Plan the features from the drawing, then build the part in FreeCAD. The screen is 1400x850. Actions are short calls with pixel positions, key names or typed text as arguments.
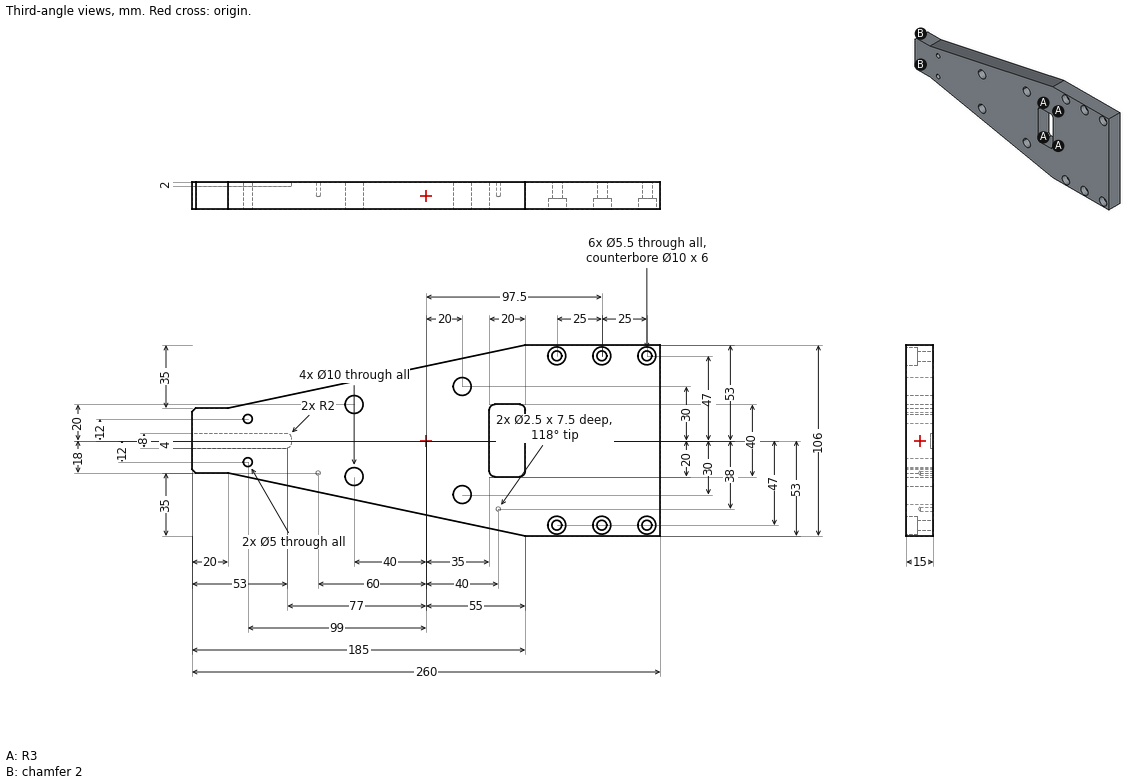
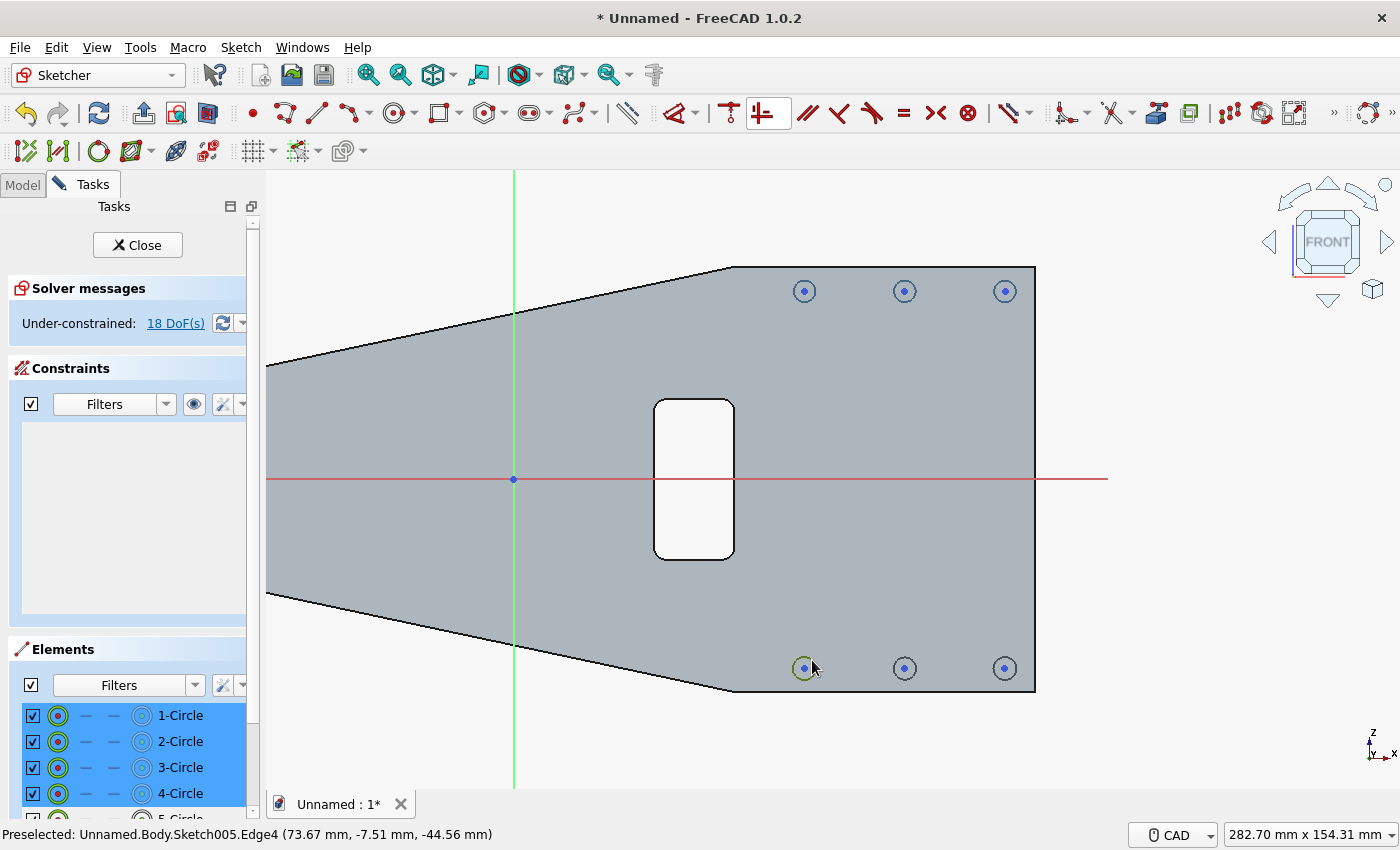
scroll(913, 661, up, 2)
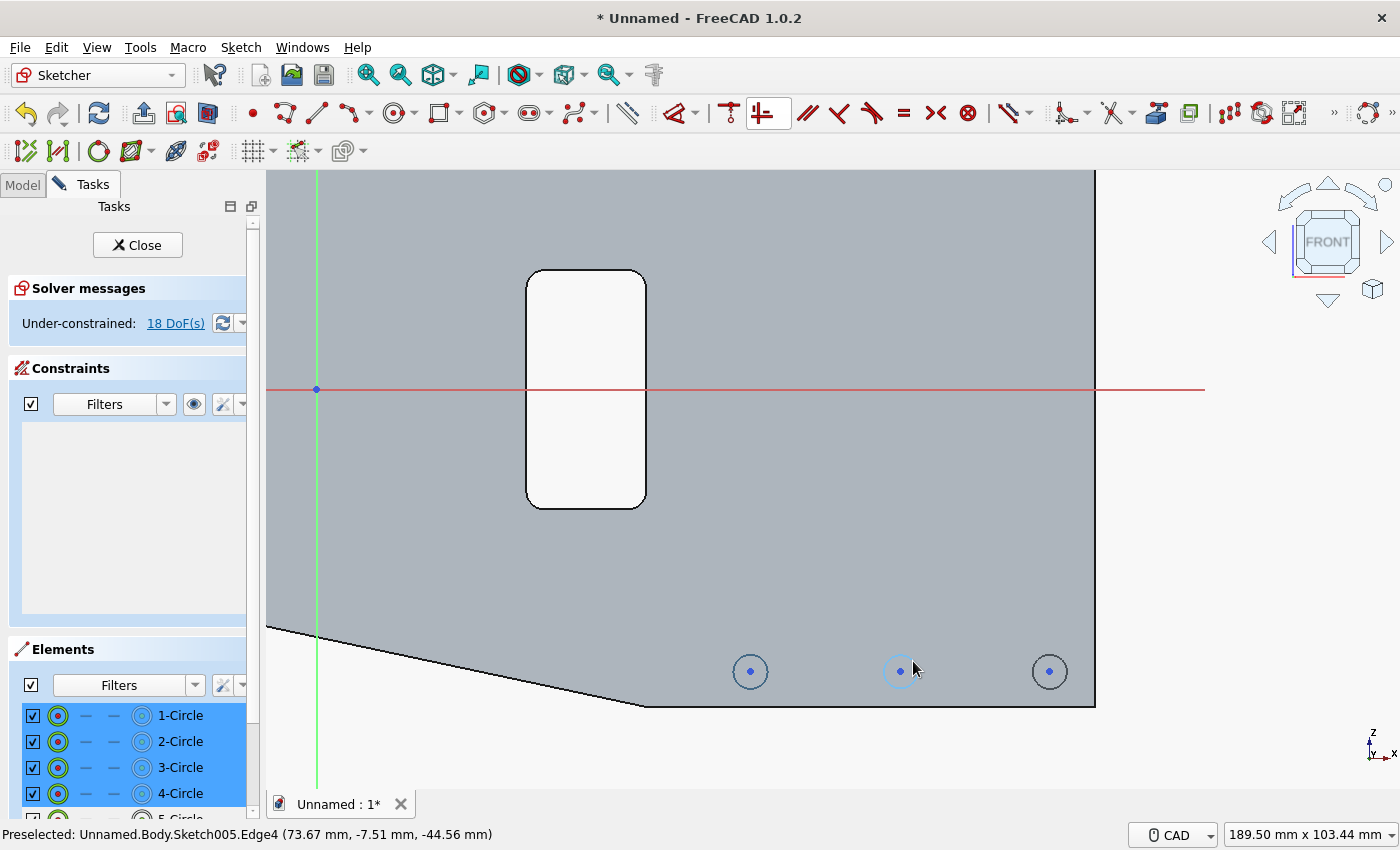
click(912, 660)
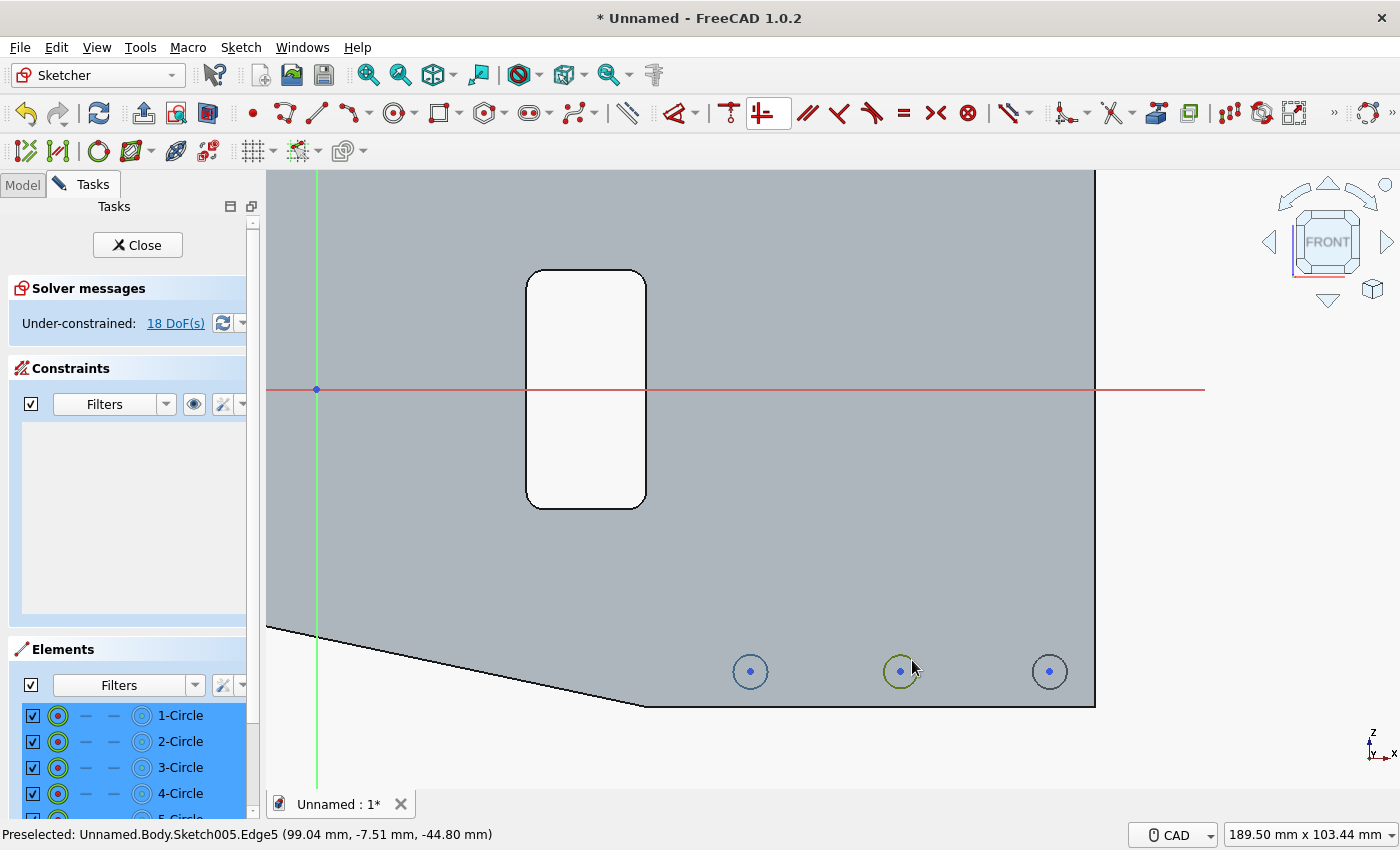
click(1062, 660)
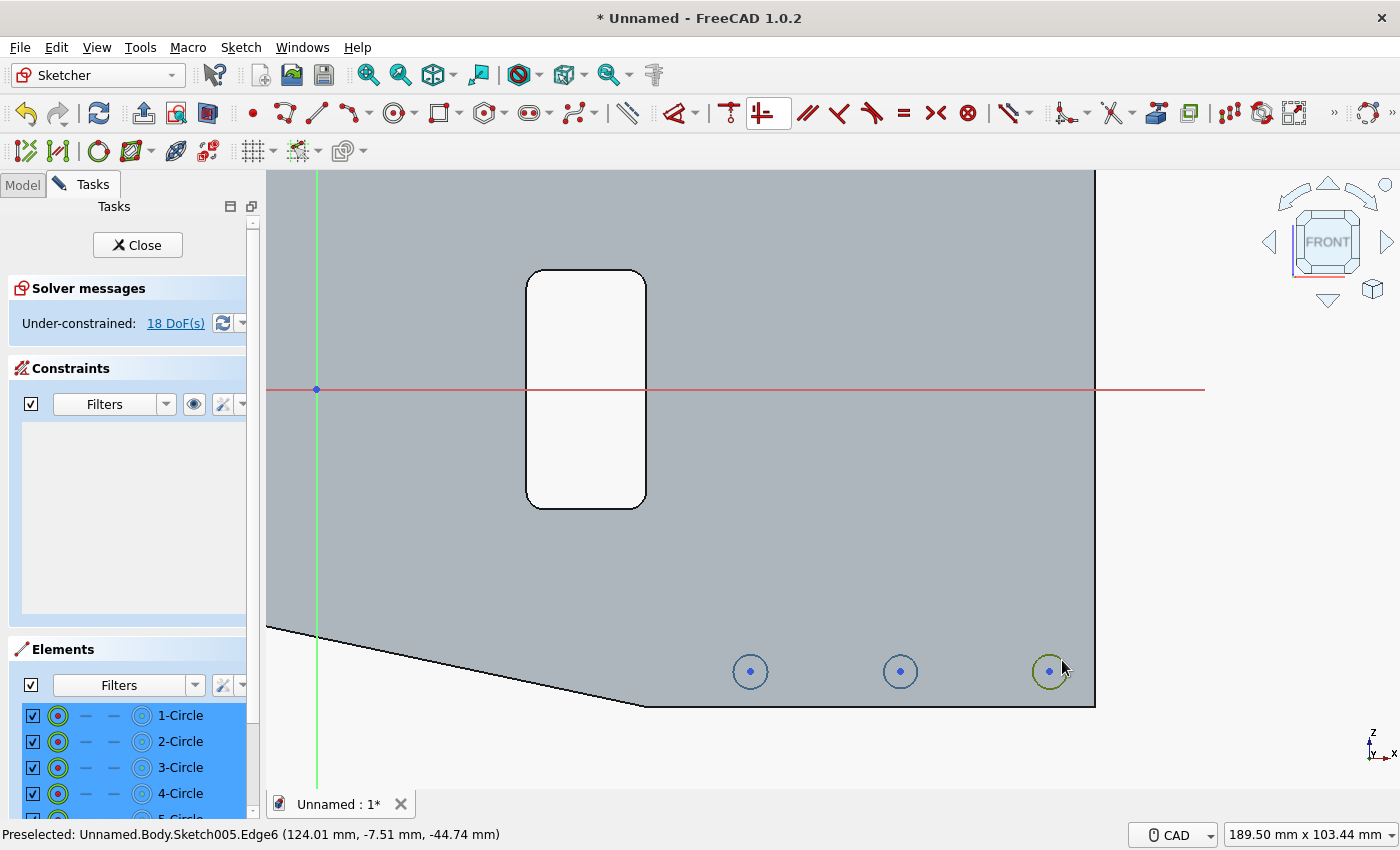
click(904, 114)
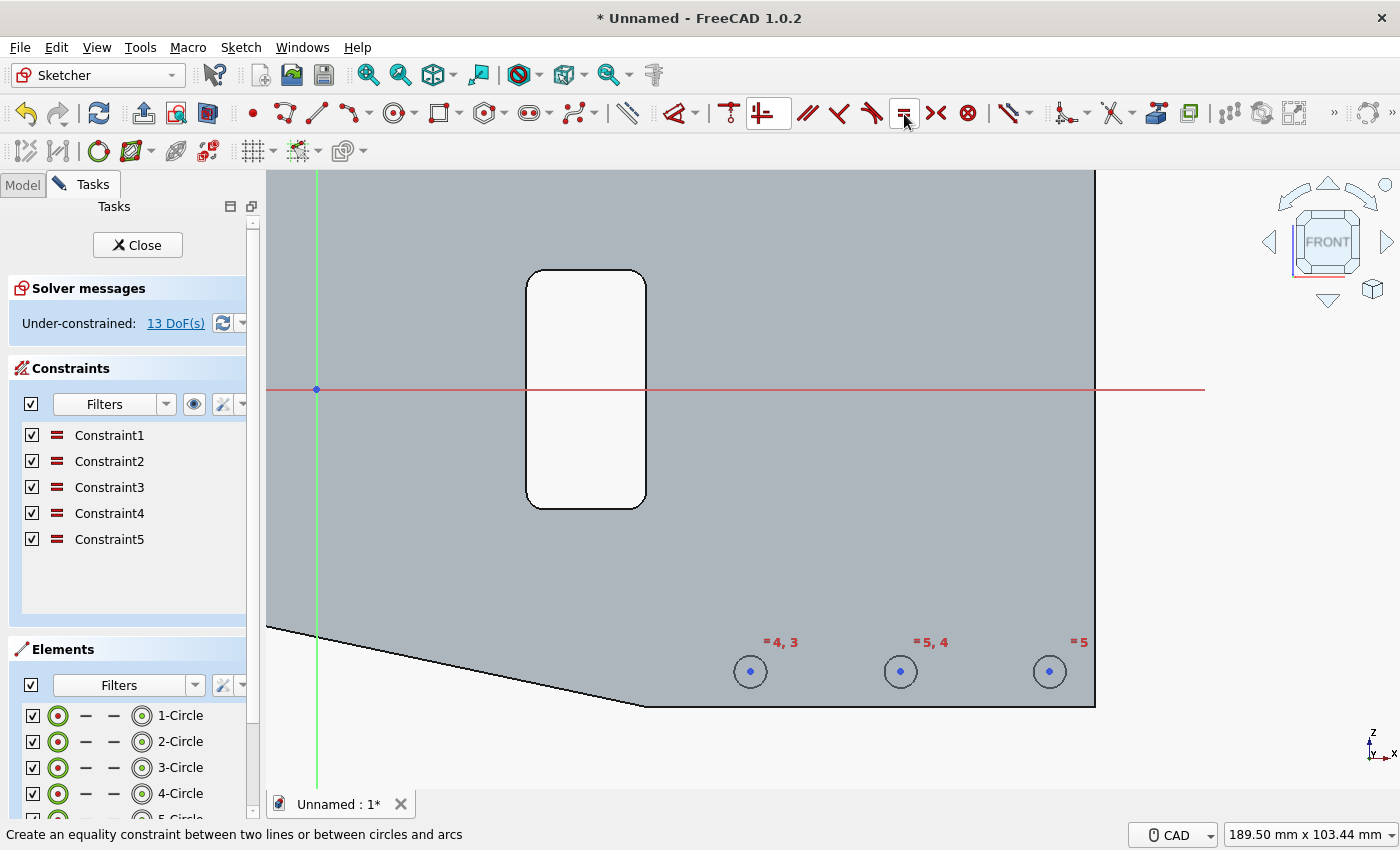
scroll(913, 662, down, 2)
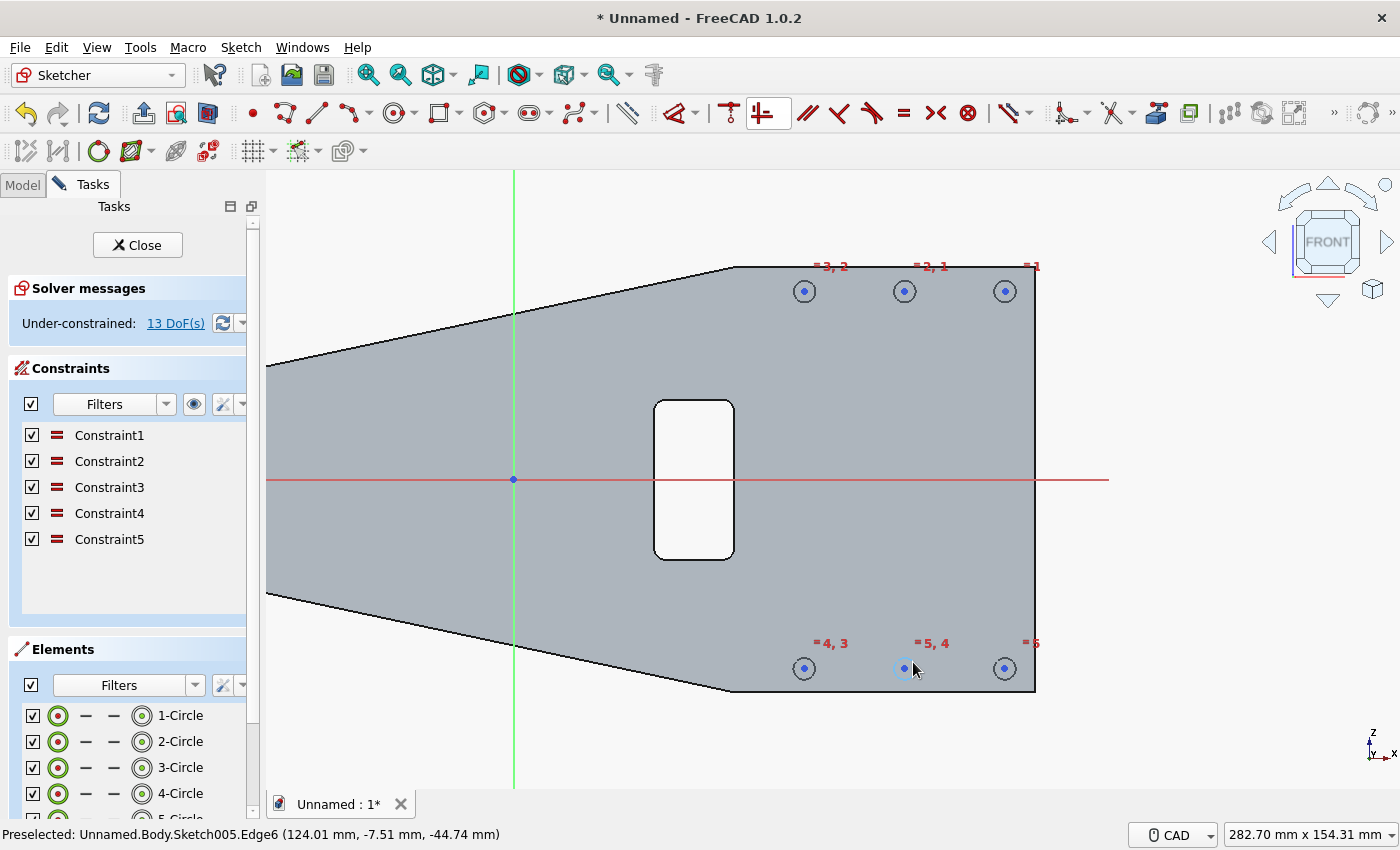
click(1005, 292)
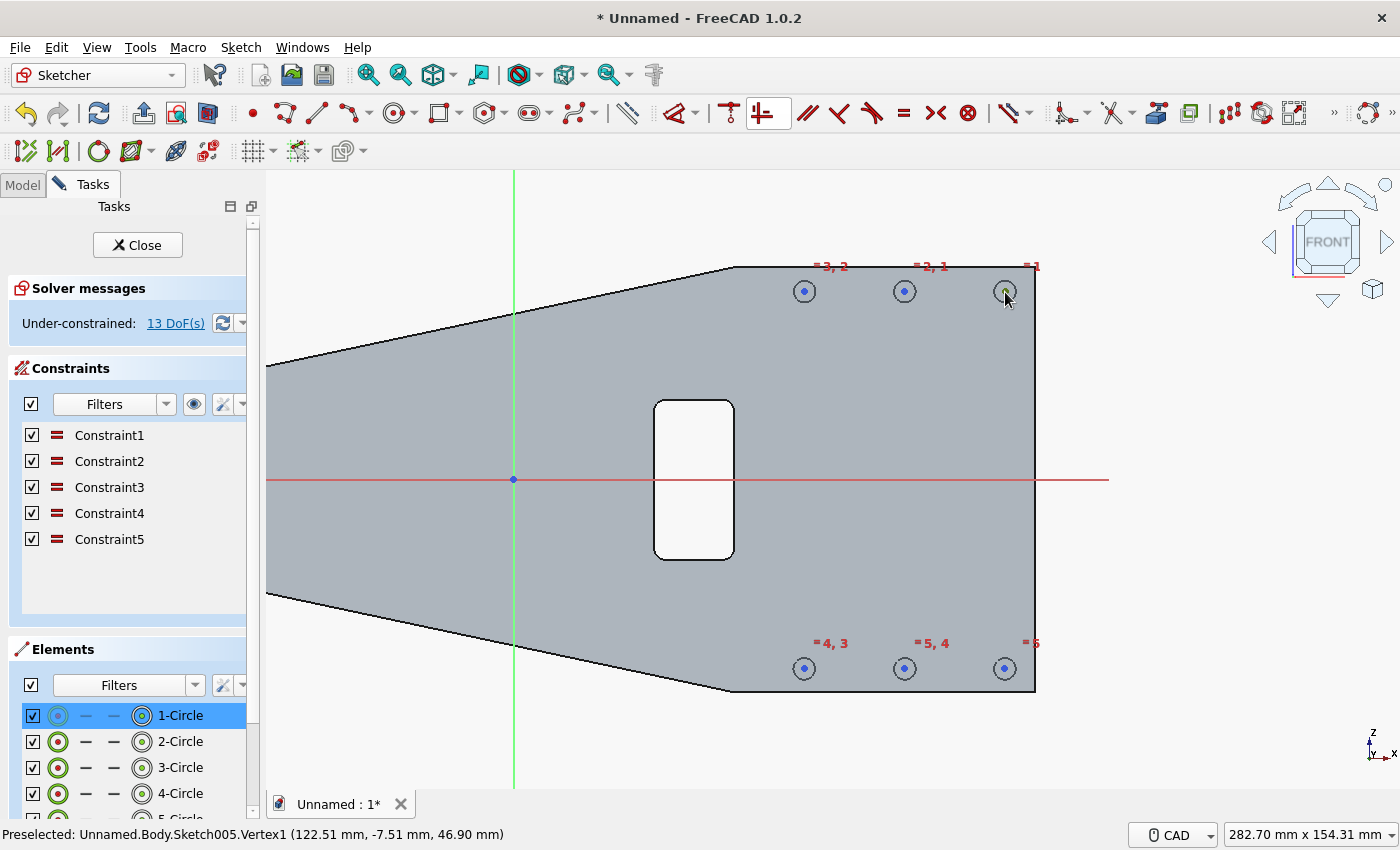
click(905, 292)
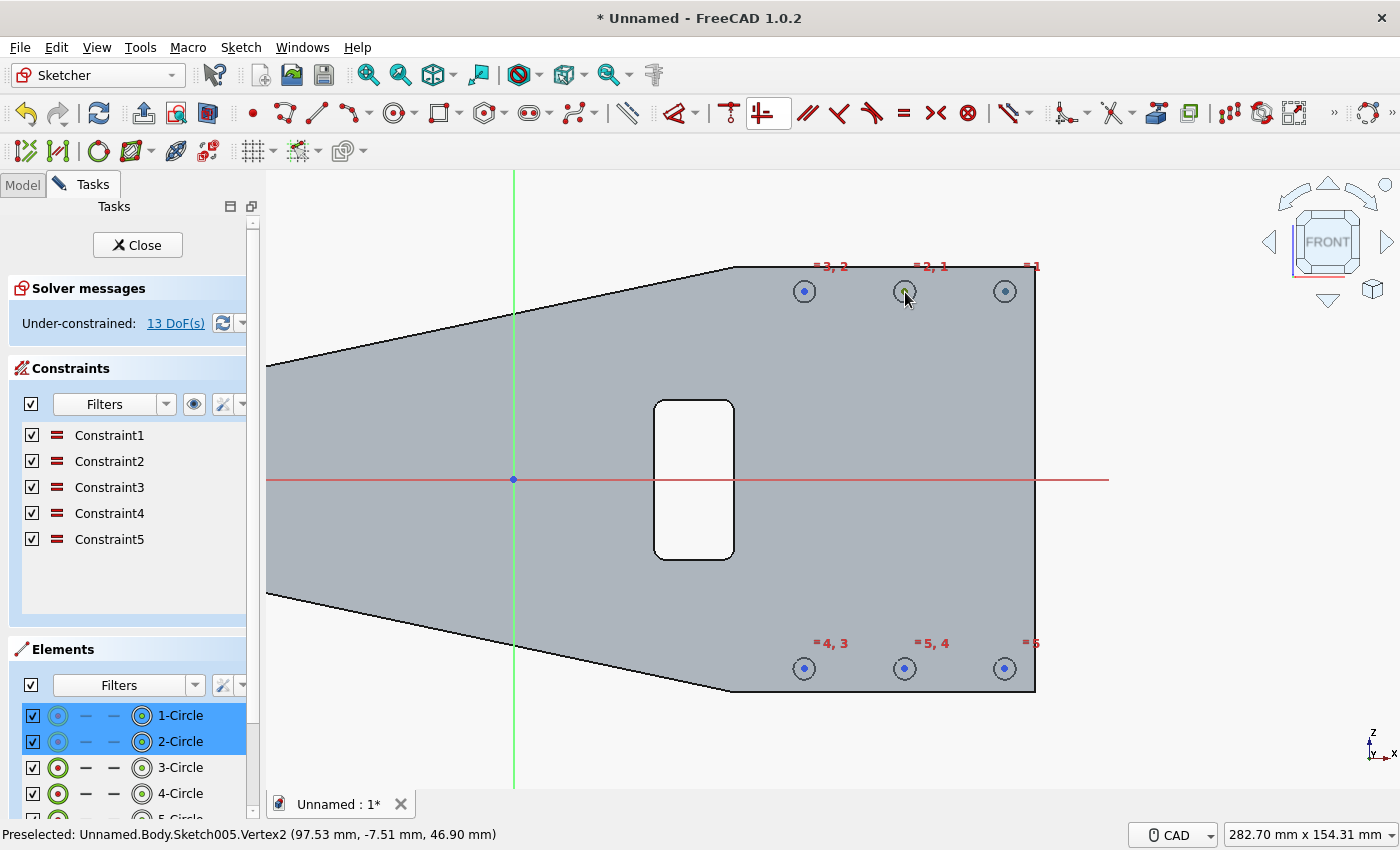
click(786, 114)